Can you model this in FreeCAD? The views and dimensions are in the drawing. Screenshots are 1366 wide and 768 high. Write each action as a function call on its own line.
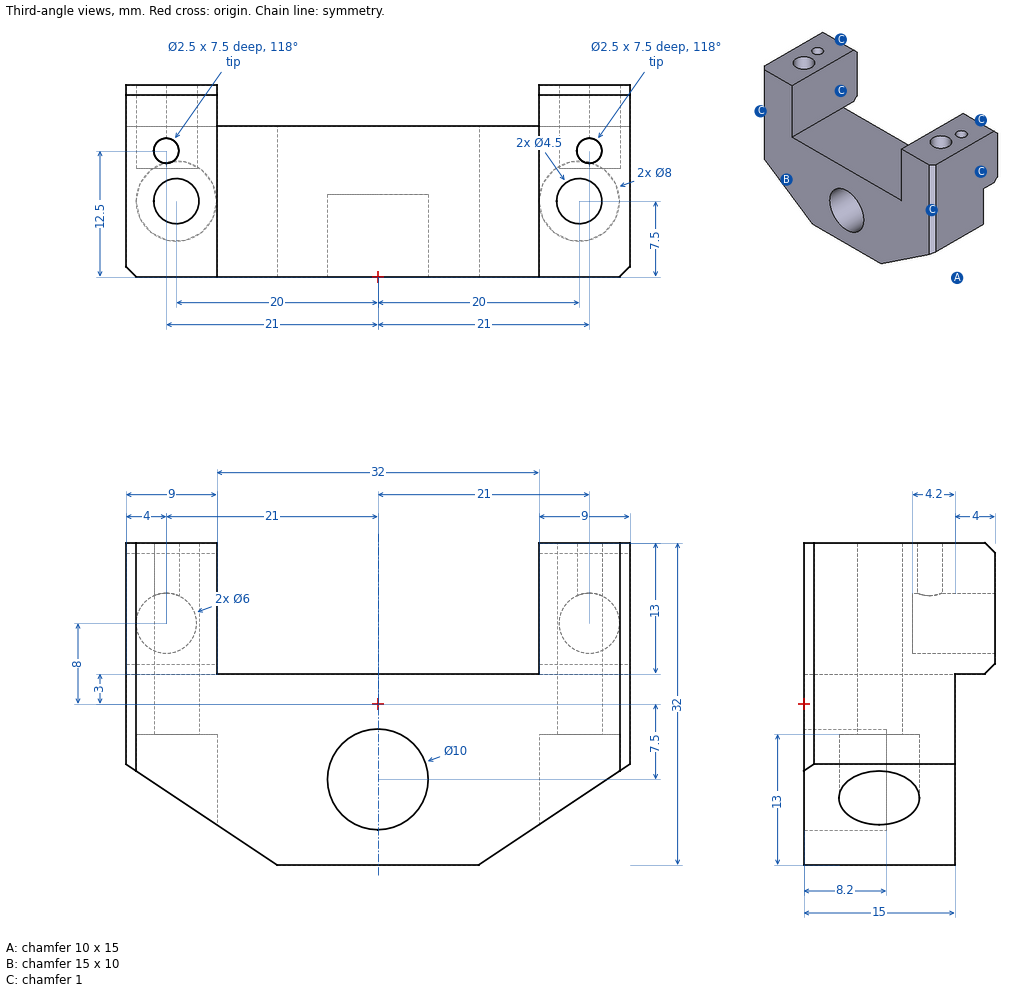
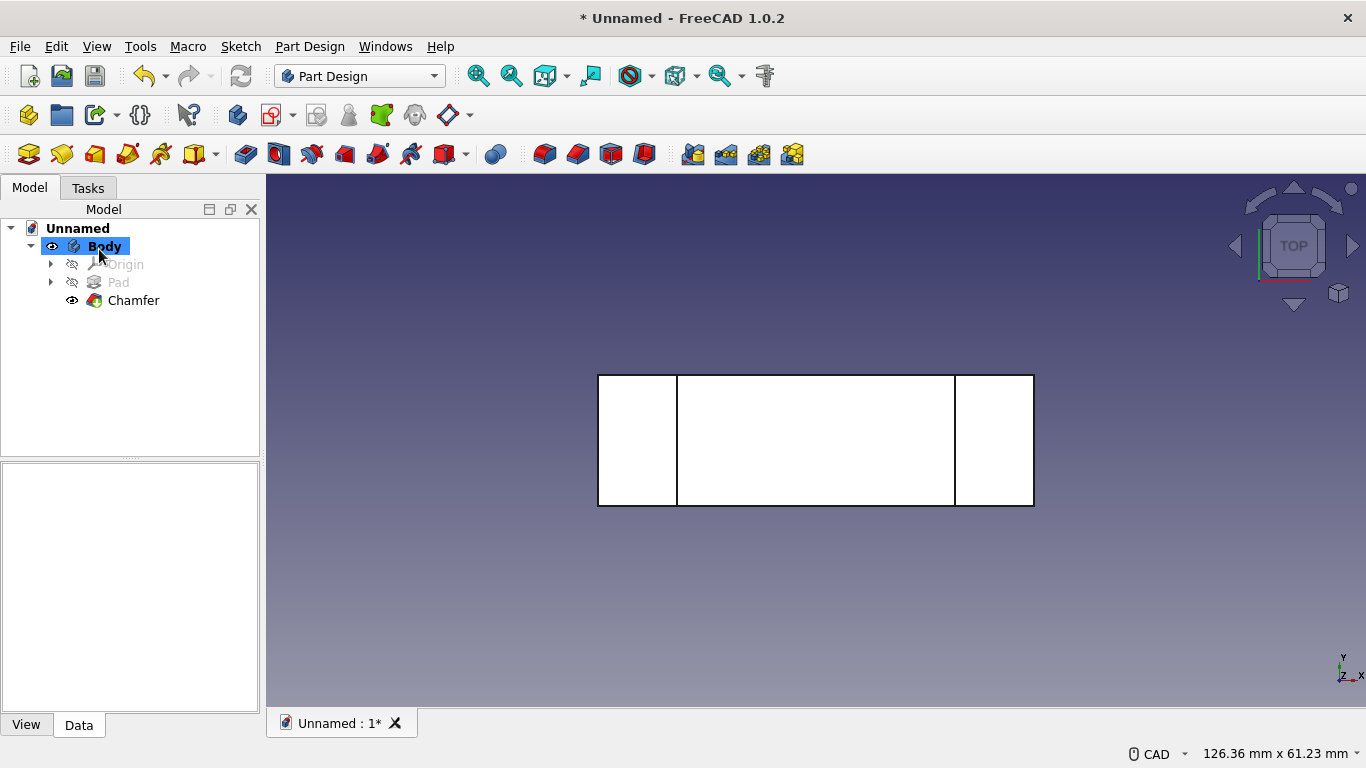
key(1)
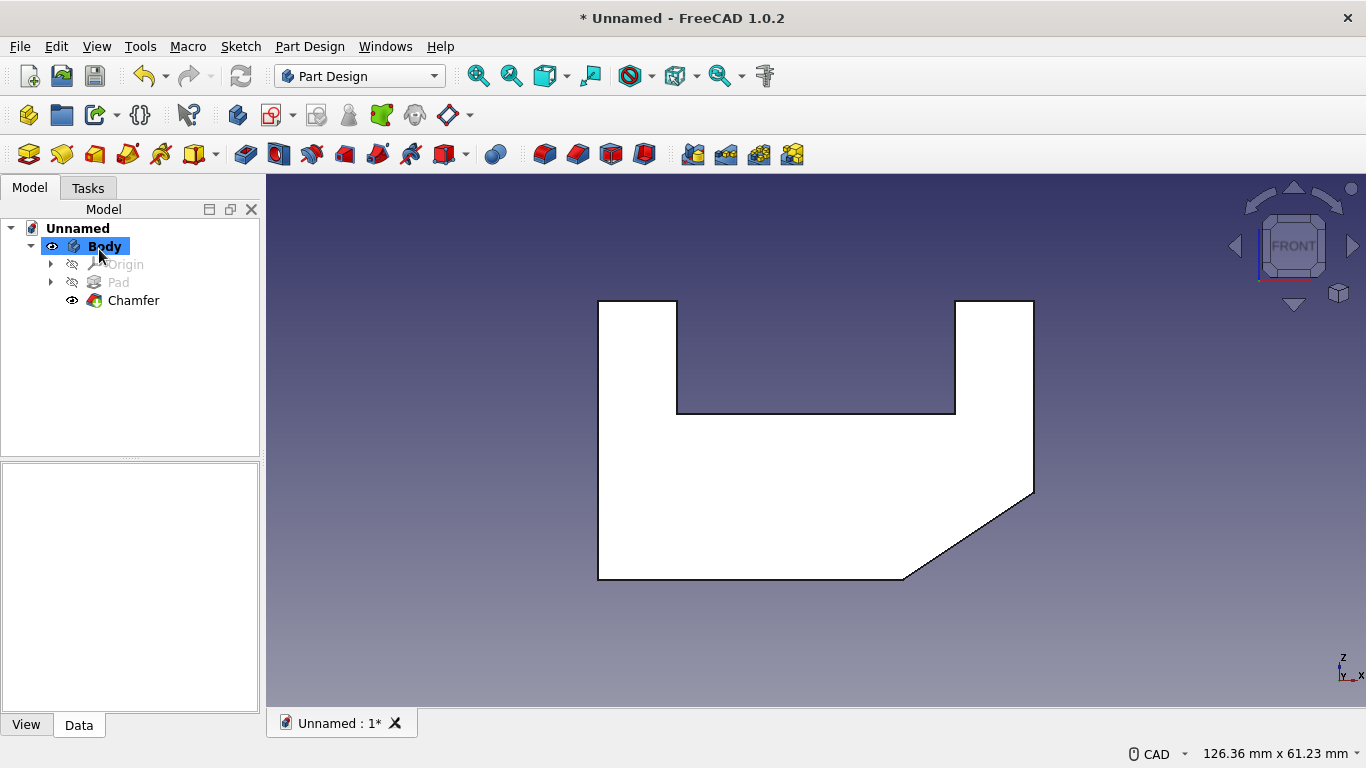
key(3)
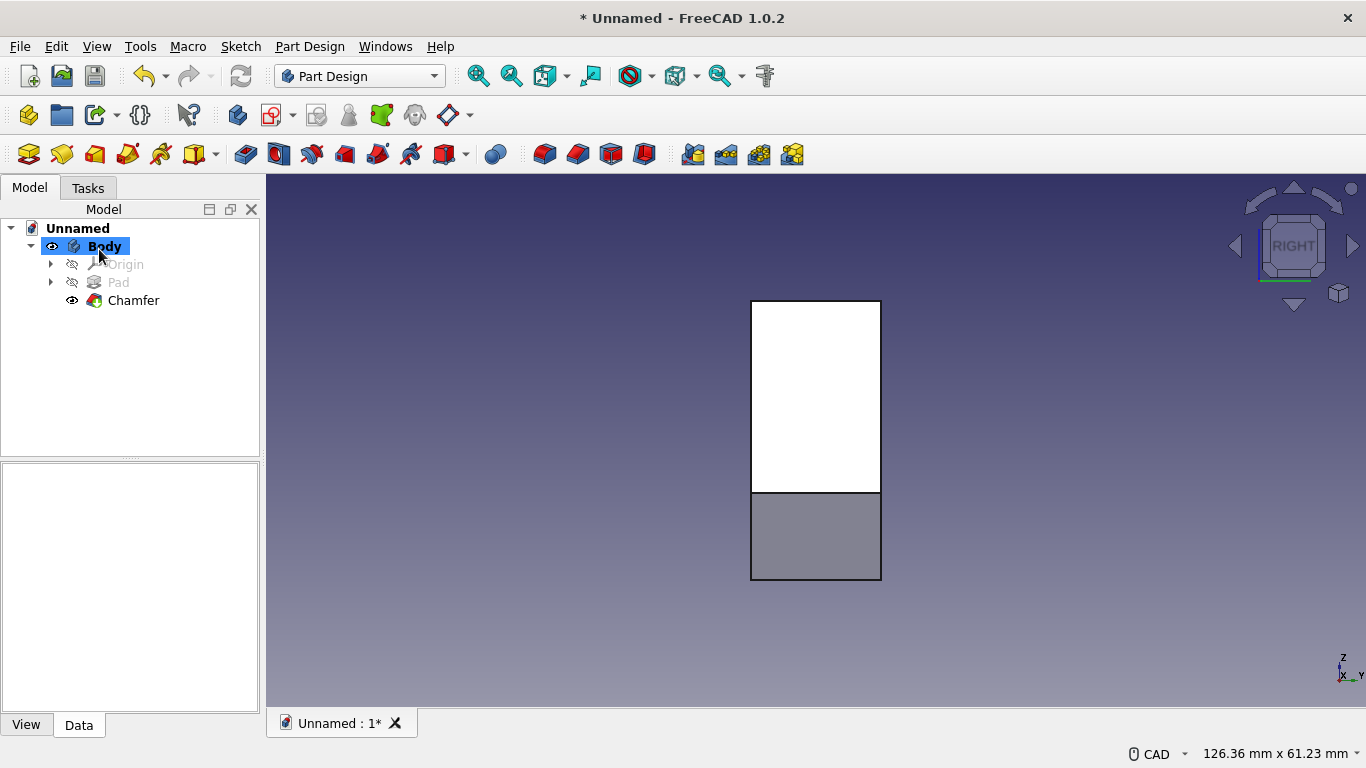
key(5)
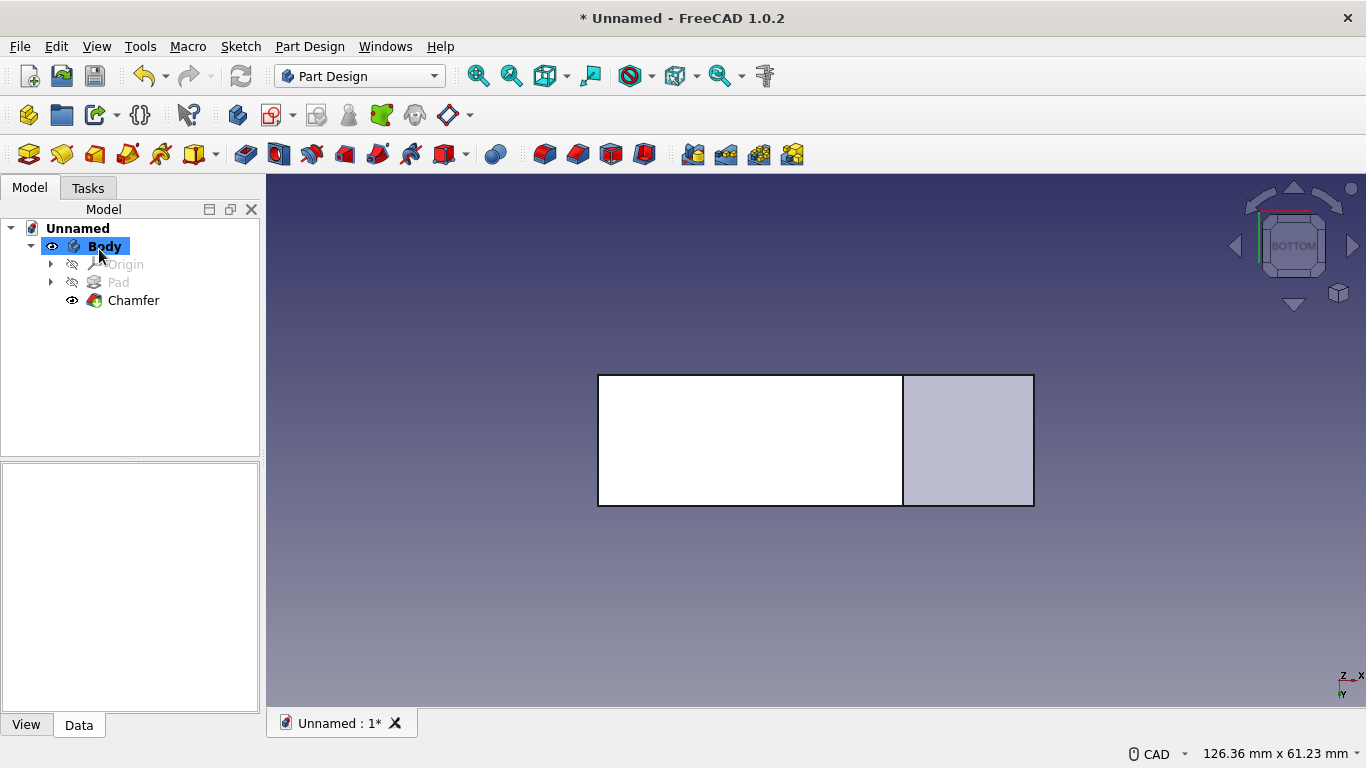
key(v)
key(f)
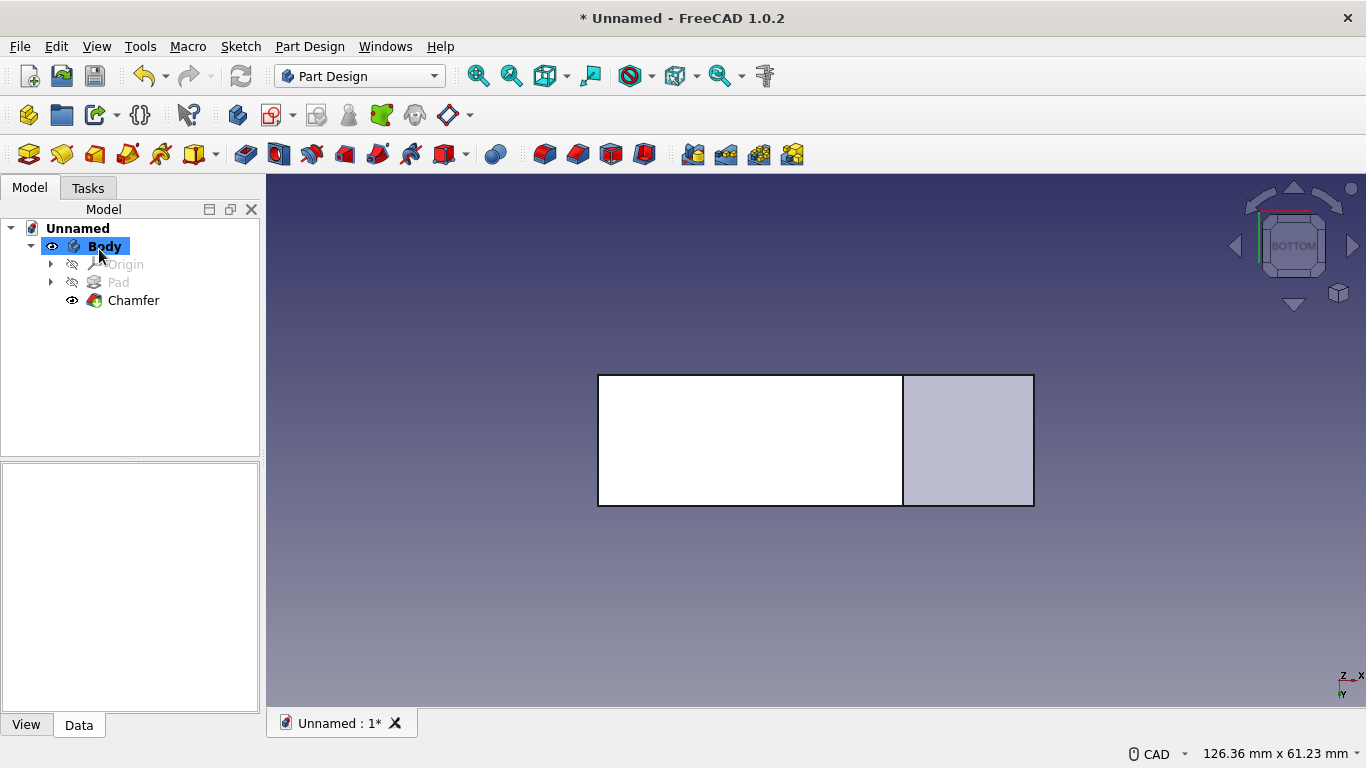
click(598, 439)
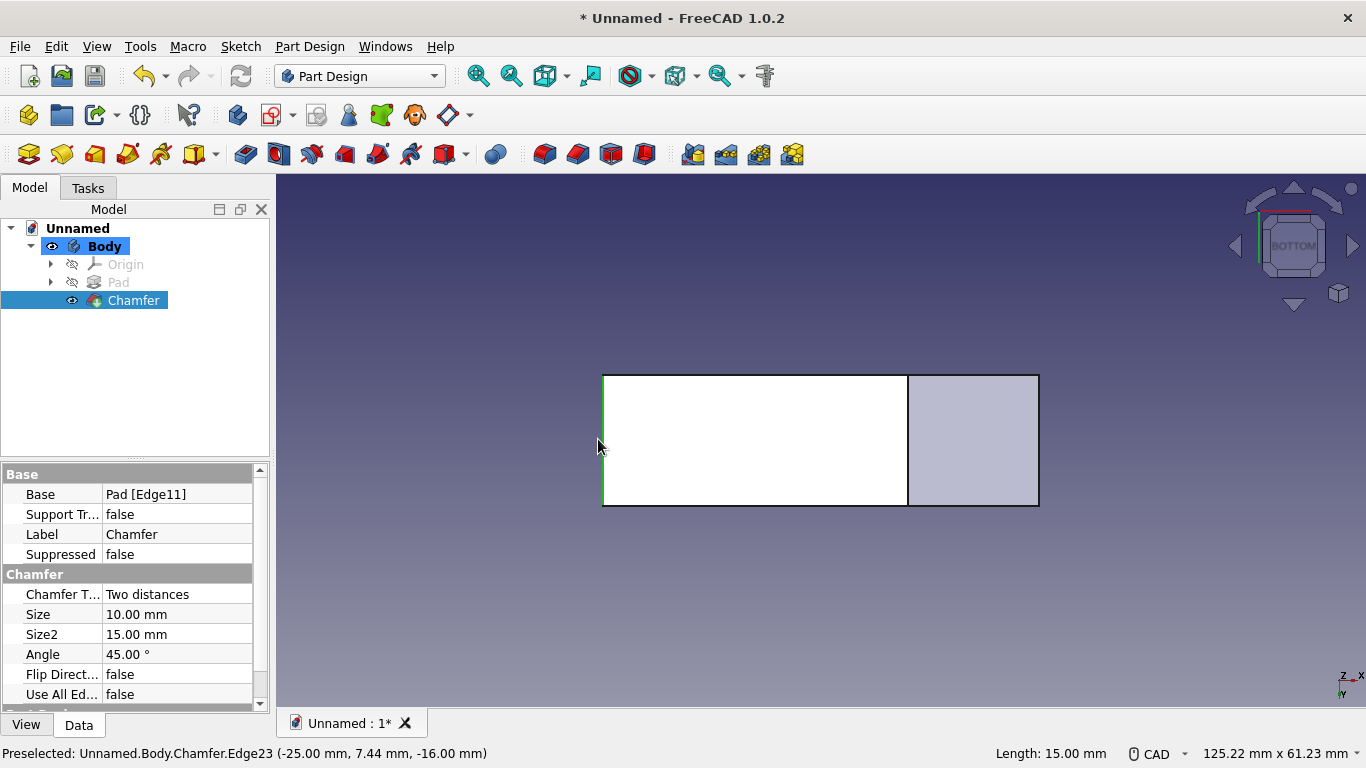
click(578, 154)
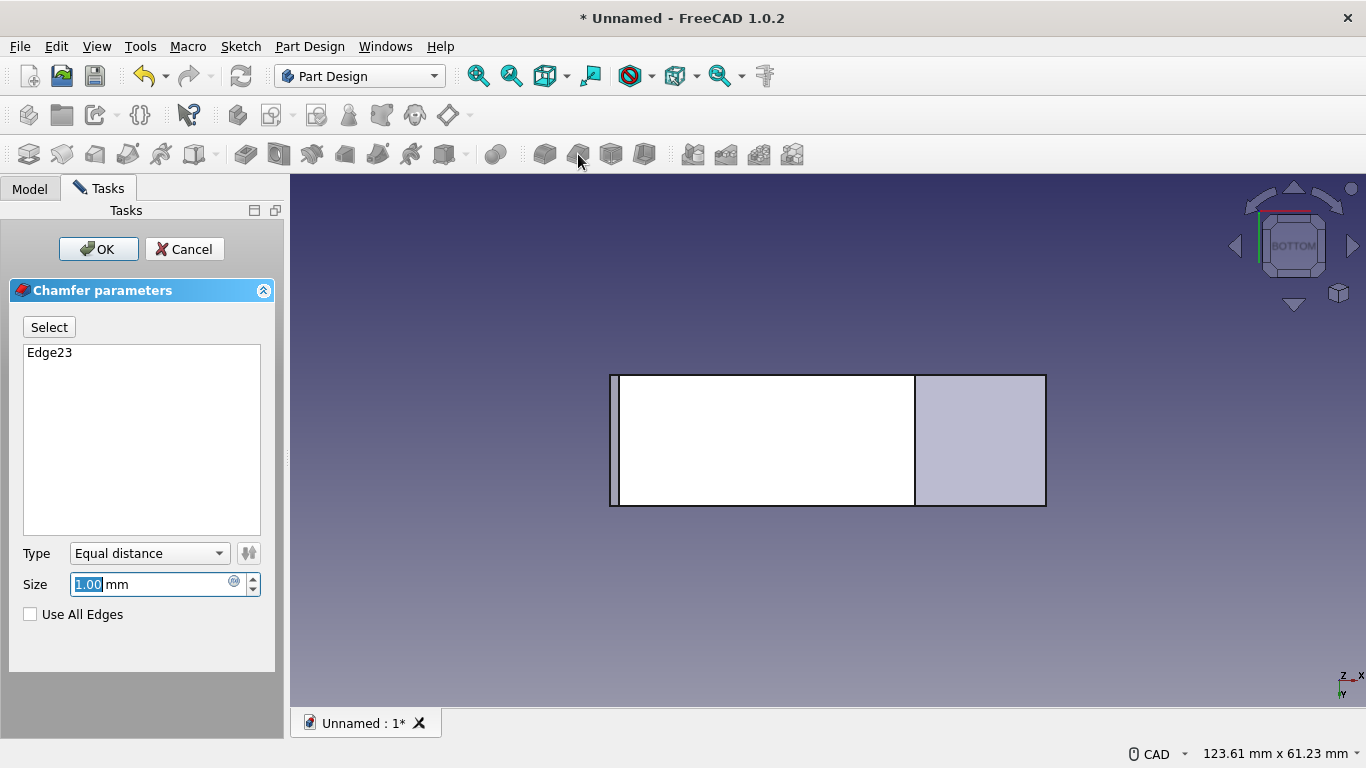
text(15)
key(Tab)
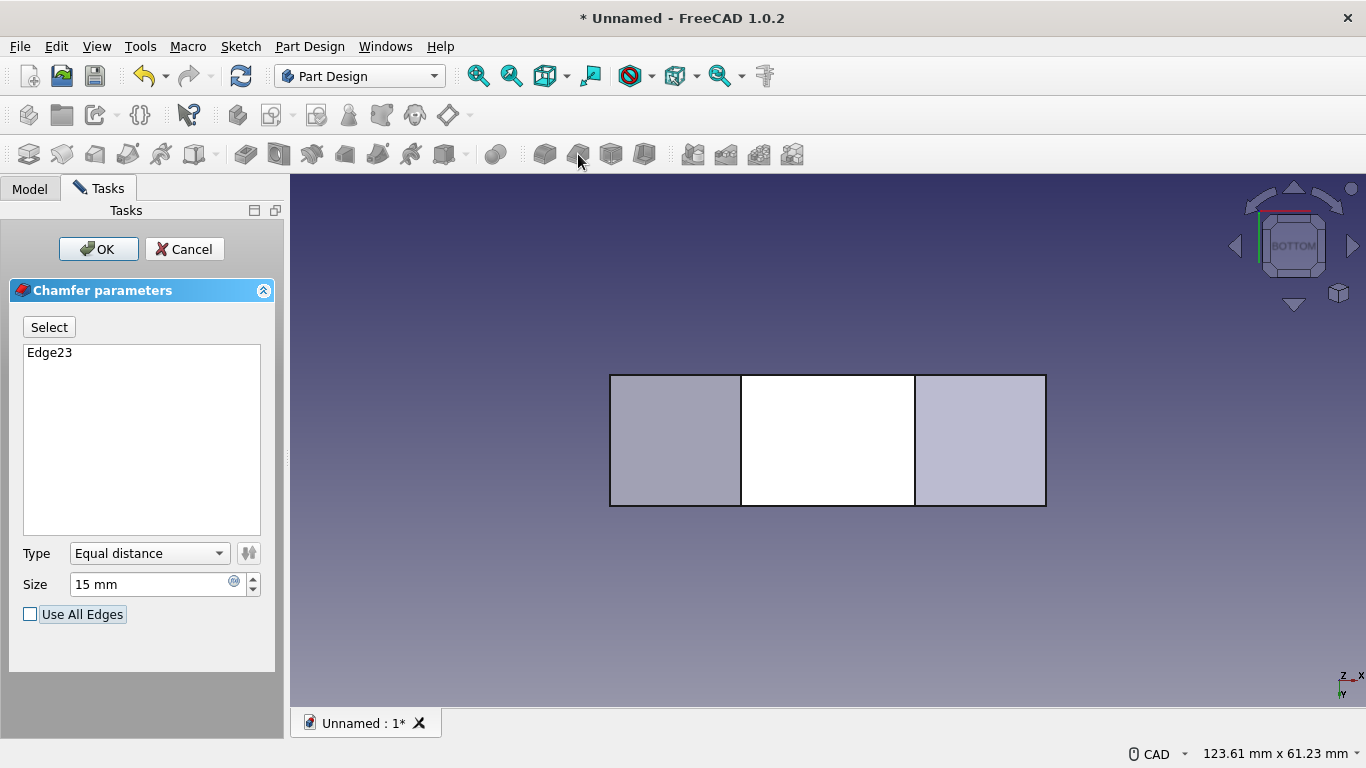
click(150, 554)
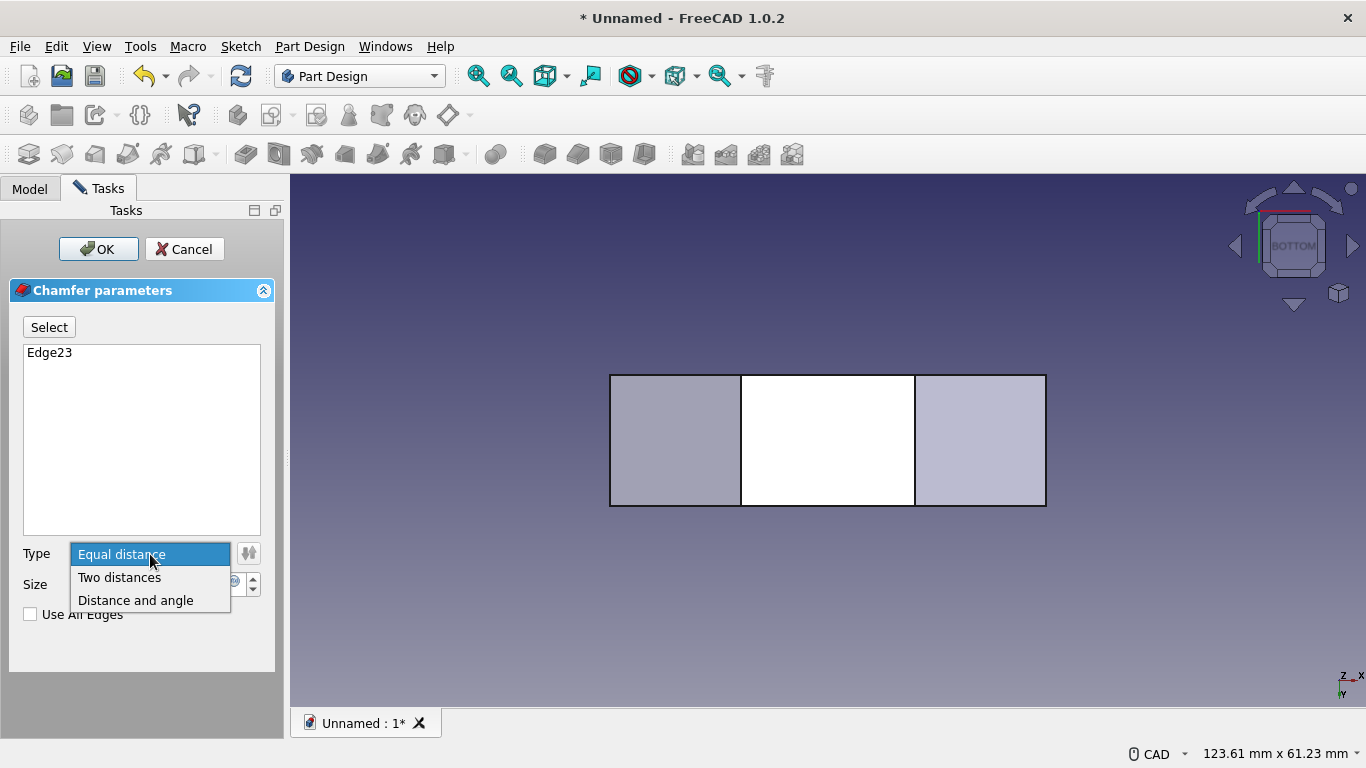
click(148, 578)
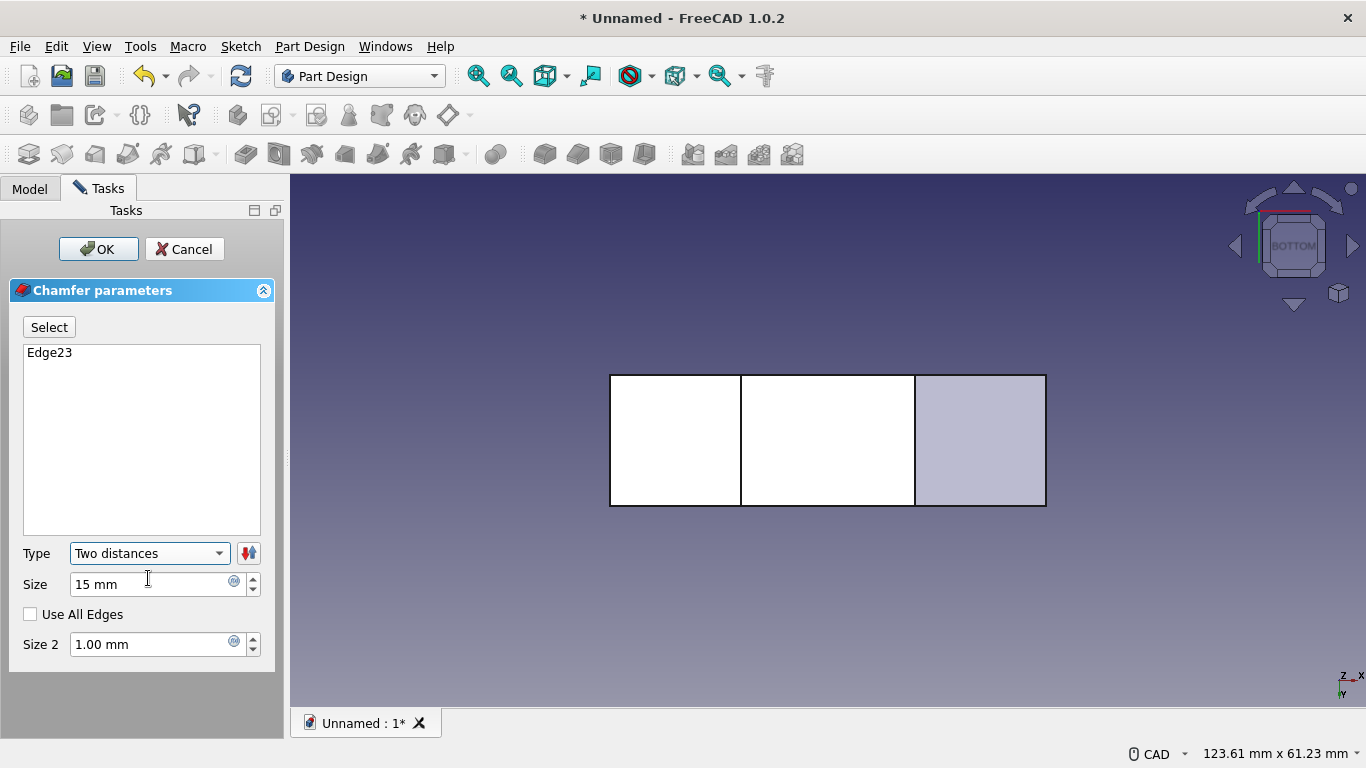
triple_click(158, 644)